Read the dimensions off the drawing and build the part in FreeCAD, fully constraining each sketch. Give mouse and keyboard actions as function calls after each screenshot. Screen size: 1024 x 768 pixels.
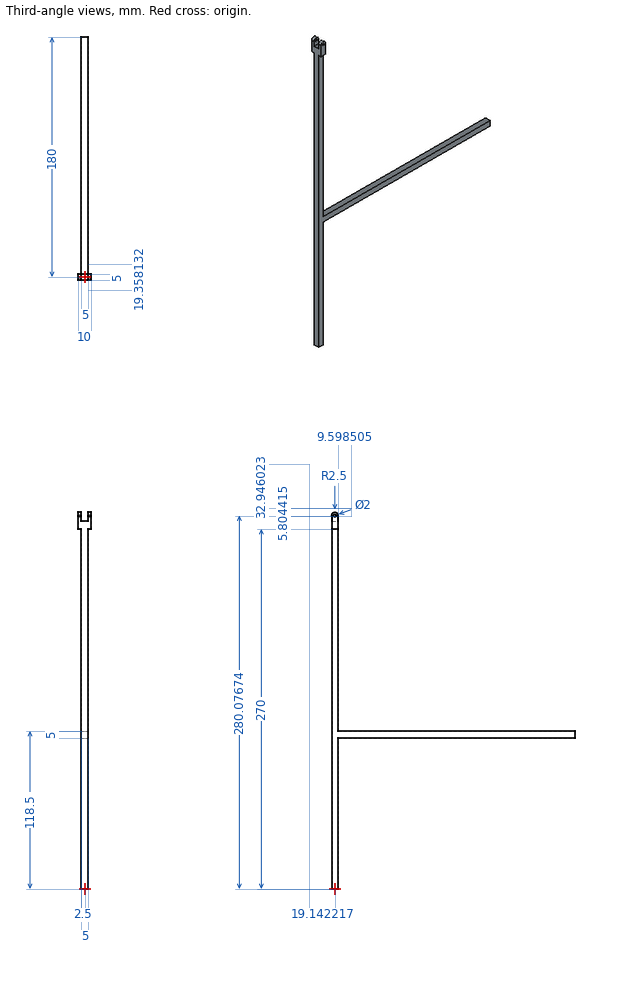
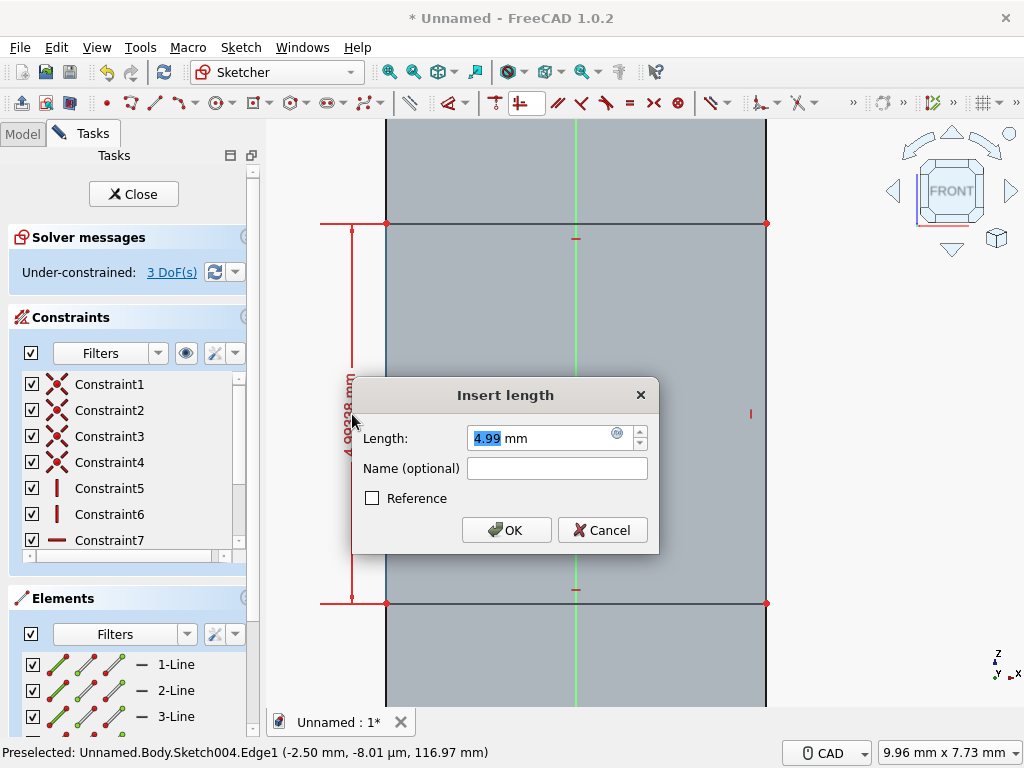
text(5)
key(Return)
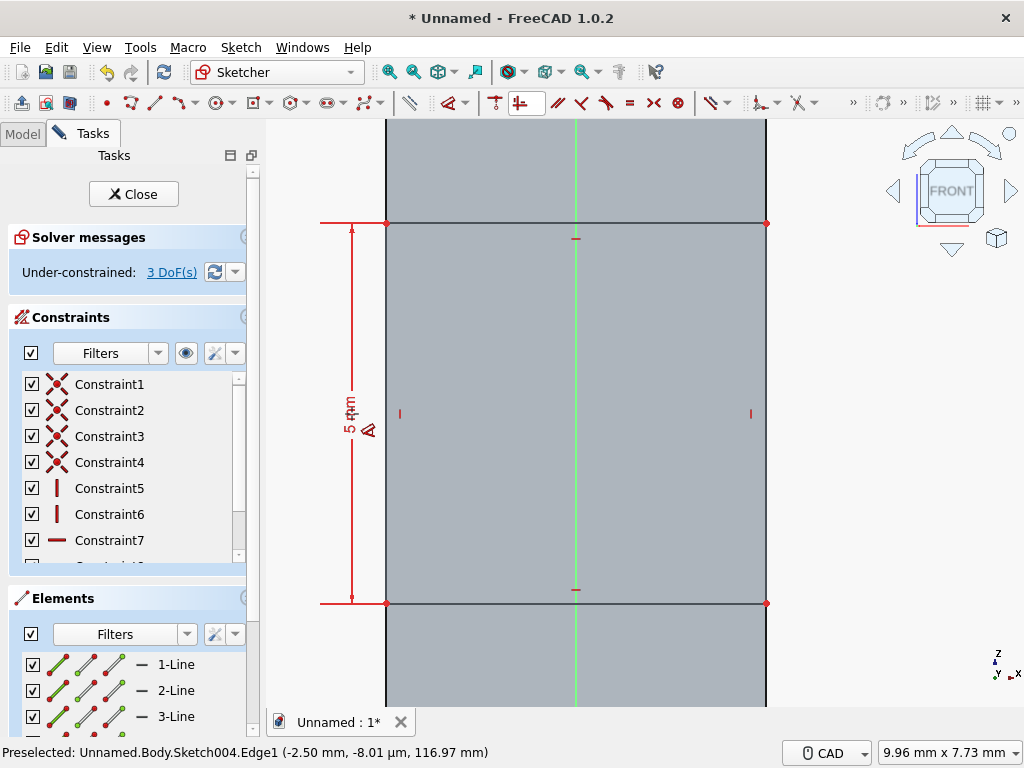
click(500, 604)
click(489, 638)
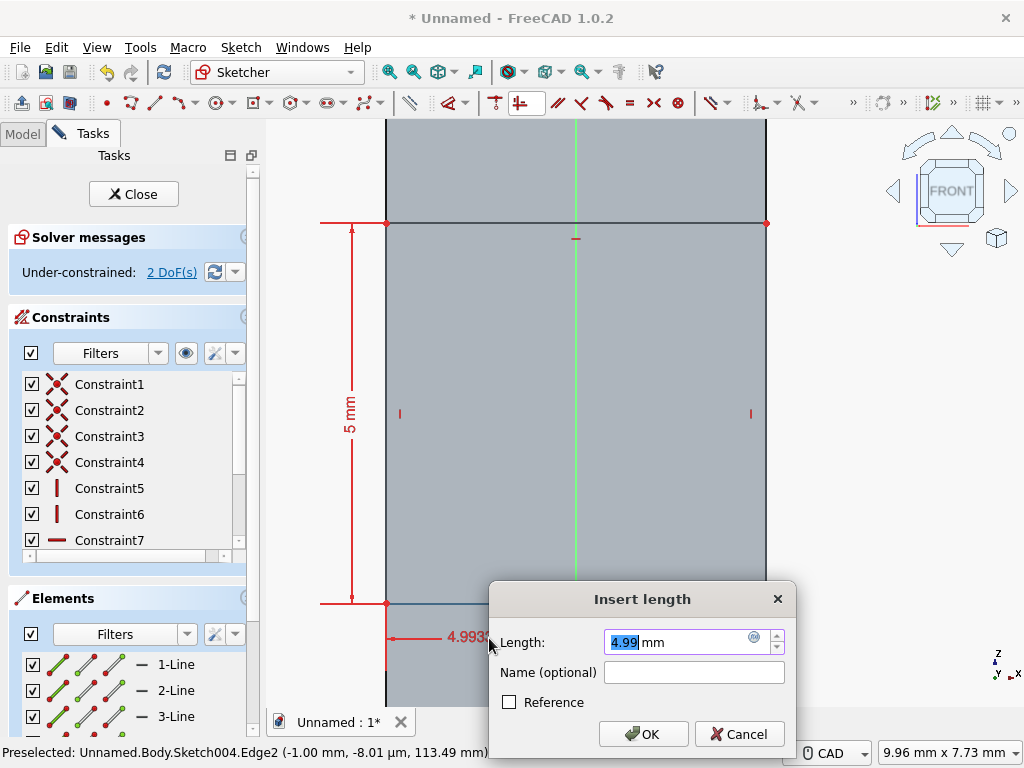
text(5)
key(Return)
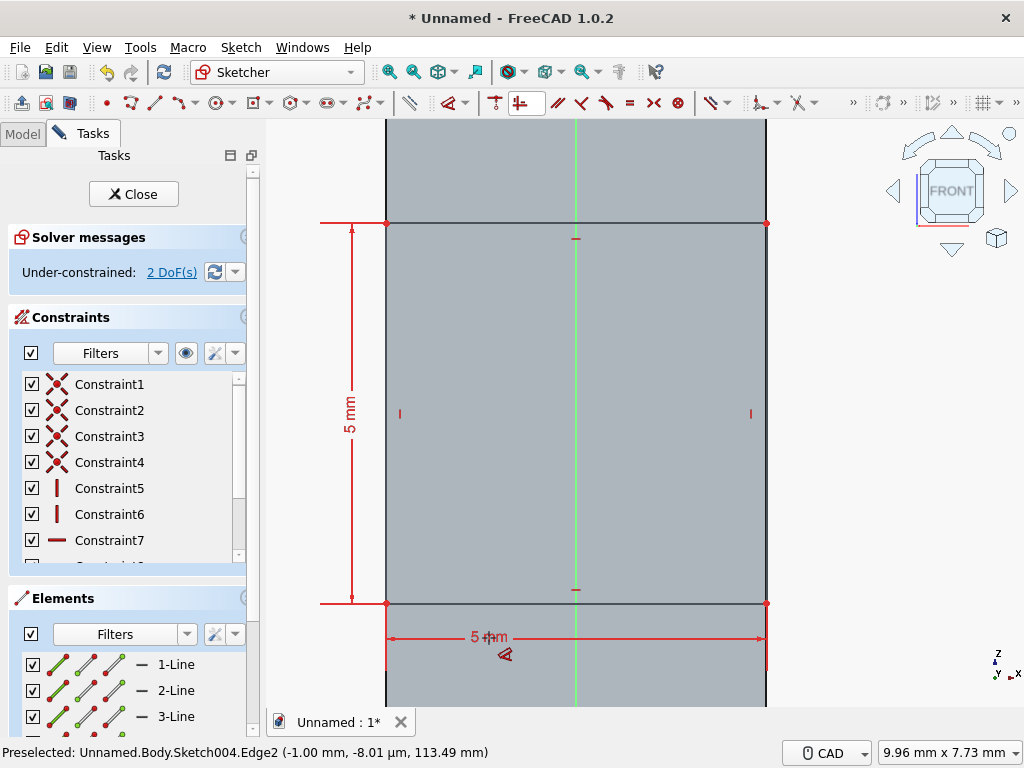
click(386, 223)
click(481, 189)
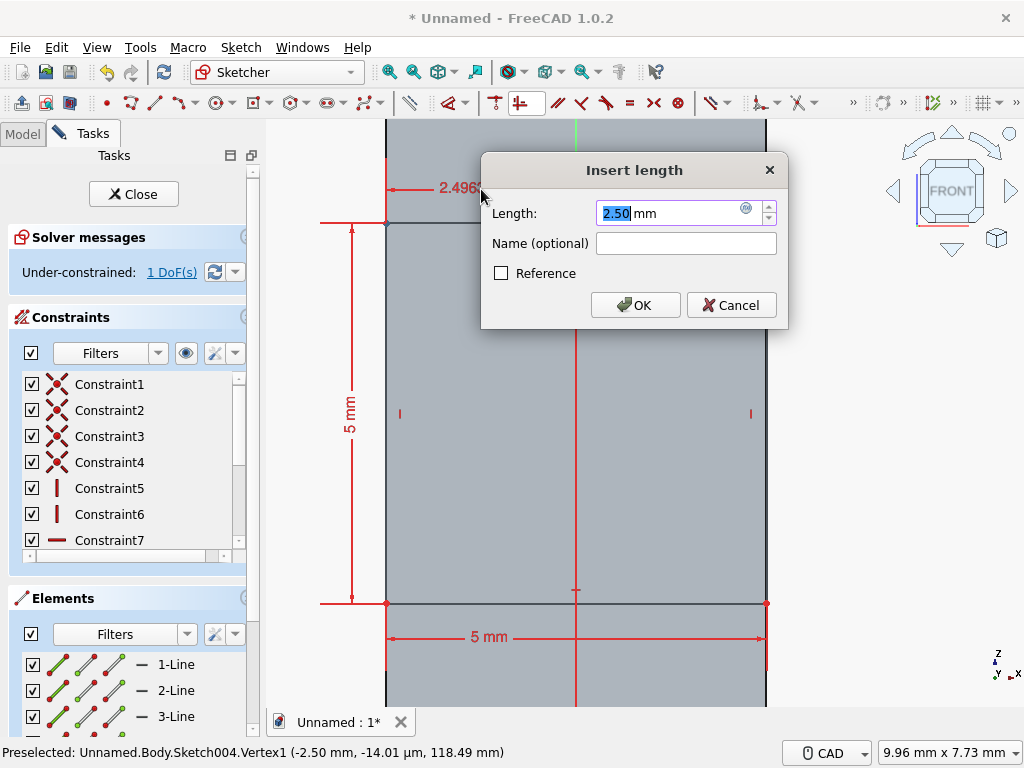
text(2.5)
key(Return)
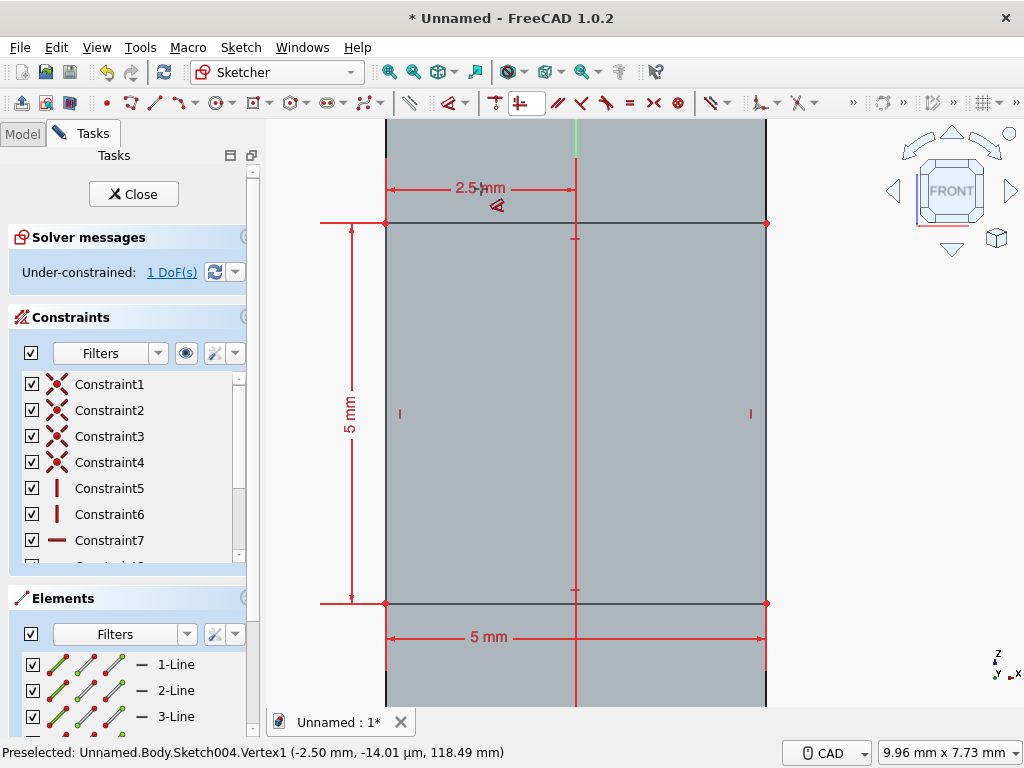
click(386, 223)
click(352, 451)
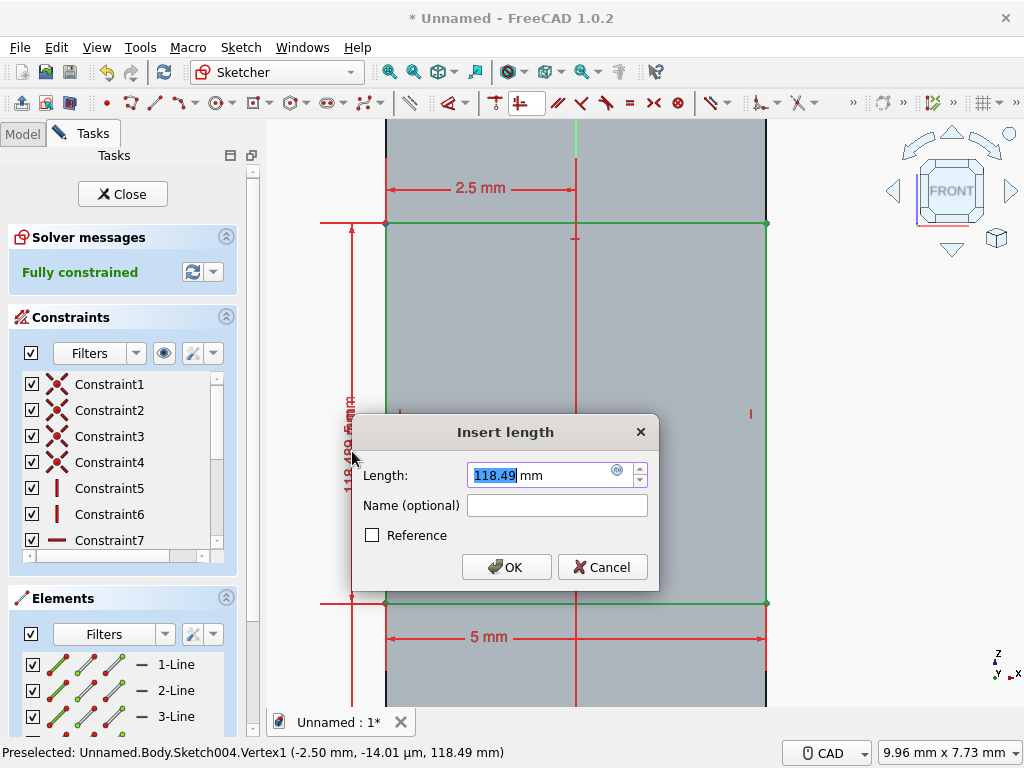
text(118.5)
key(Return)
key(Escape)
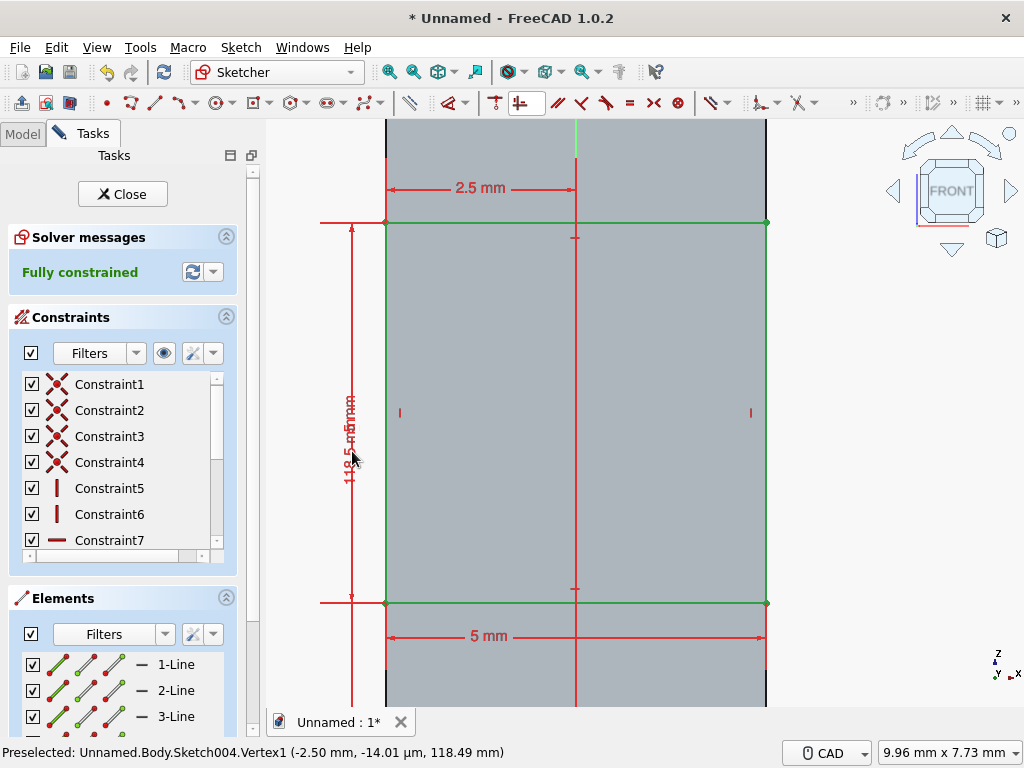
click(123, 194)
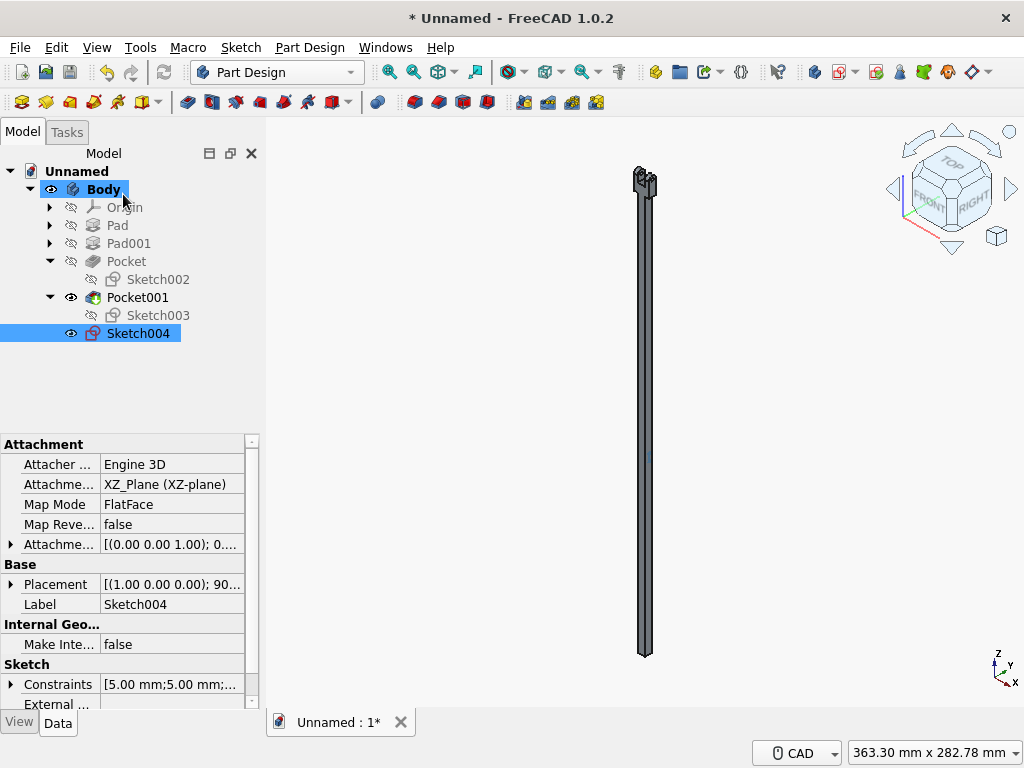
click(22, 102)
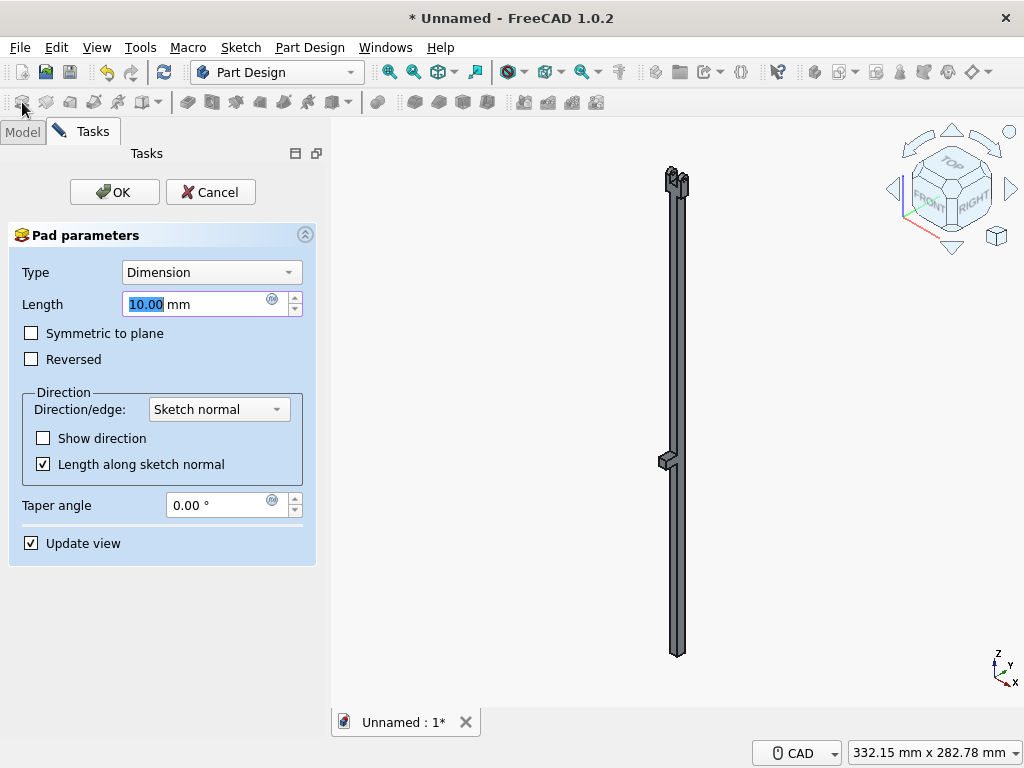
text(180)
key(Tab)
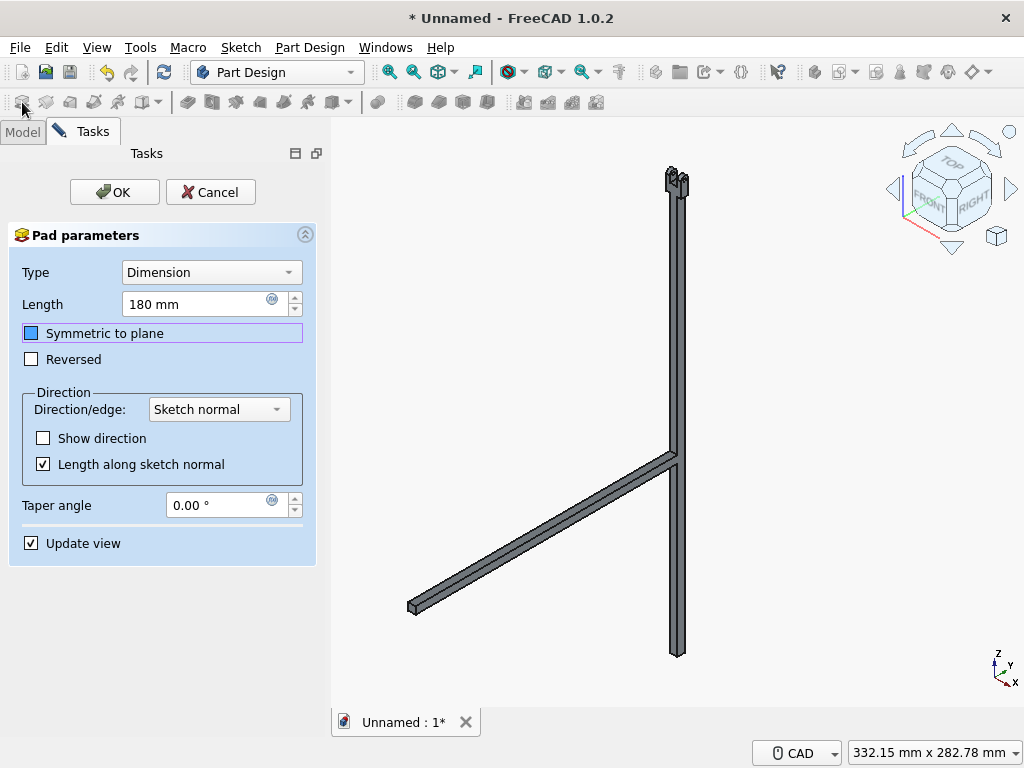
click(30, 359)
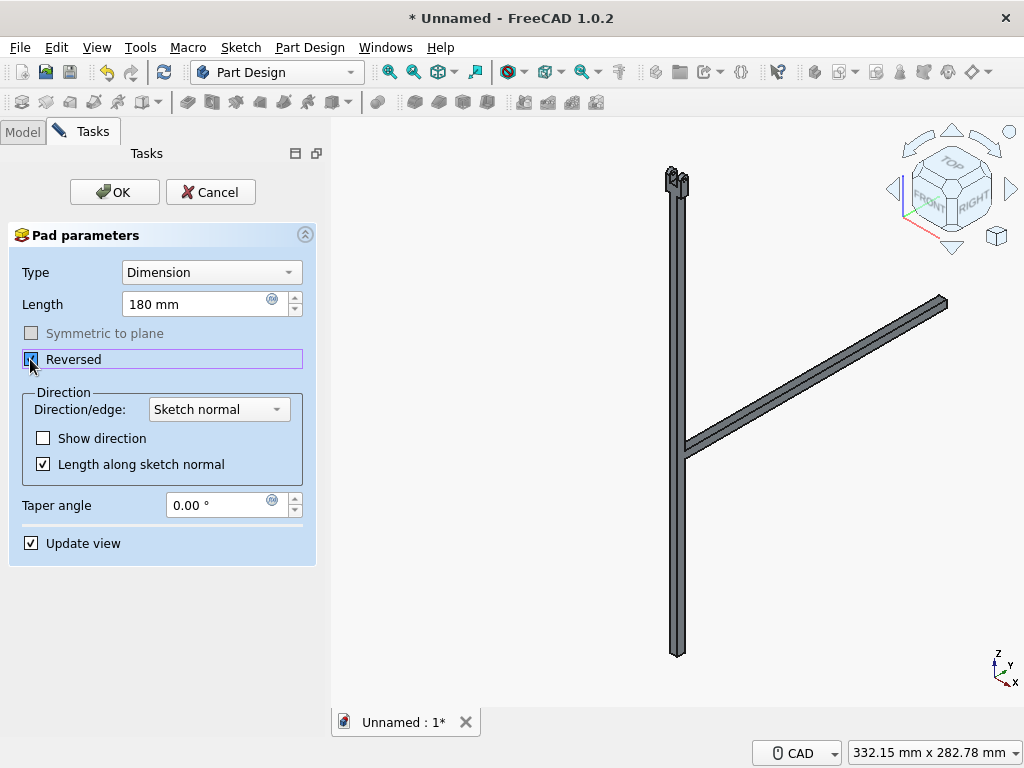
click(115, 192)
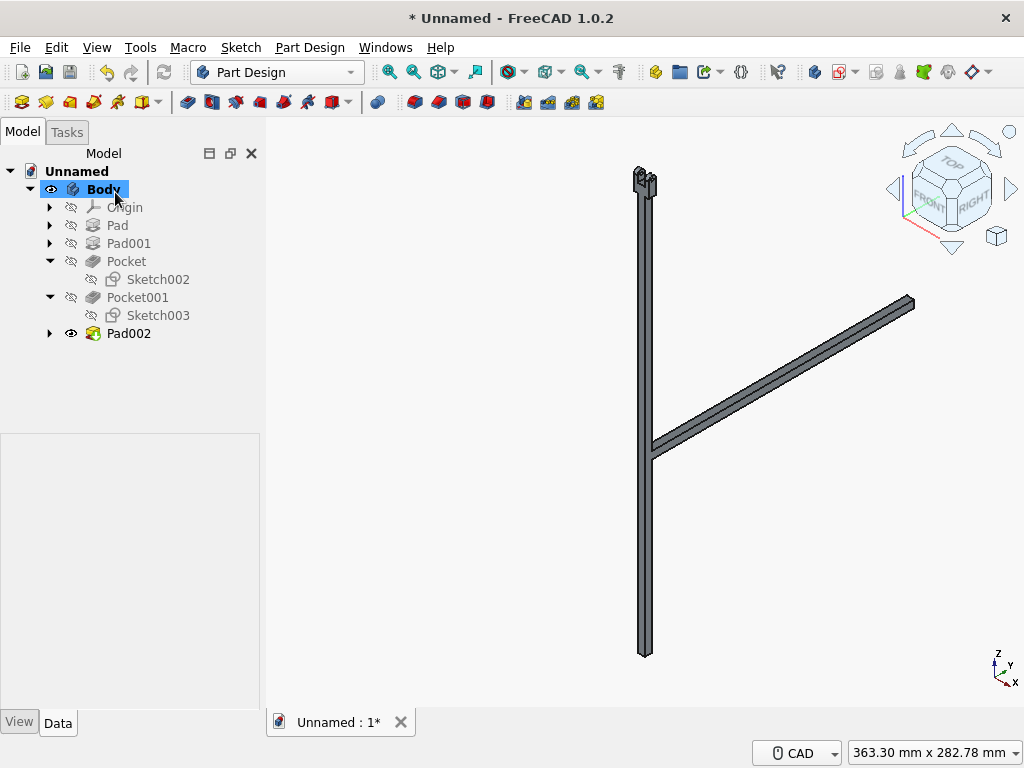
click(390, 72)